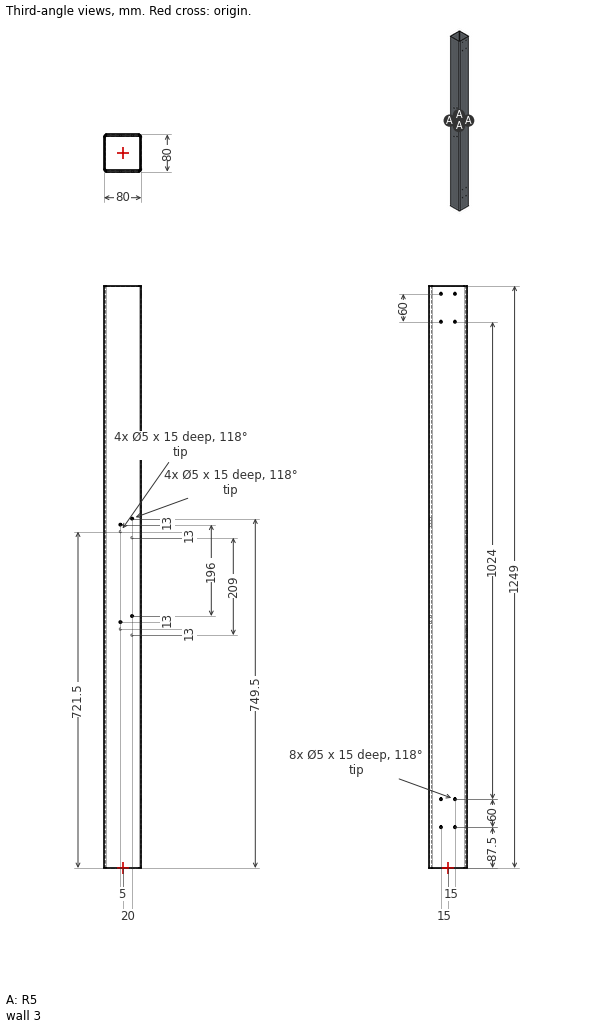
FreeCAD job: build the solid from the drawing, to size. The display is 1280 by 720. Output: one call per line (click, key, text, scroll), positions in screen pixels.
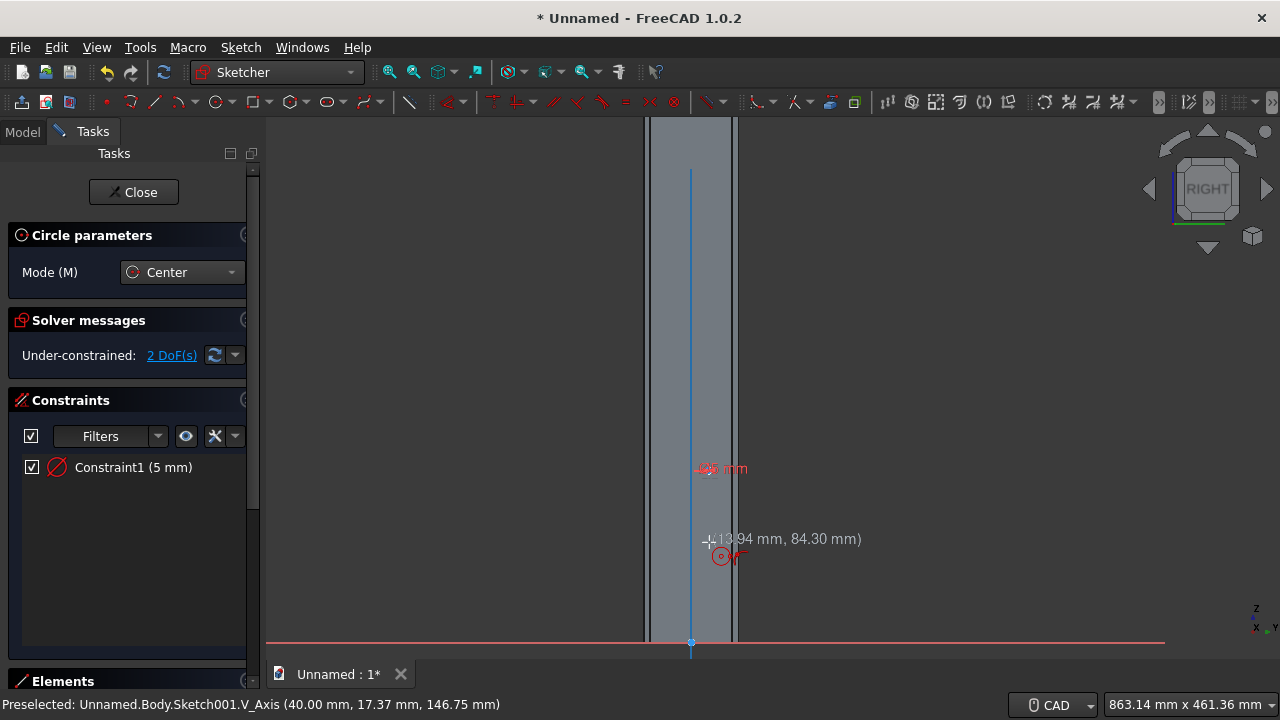
click(709, 540)
move(711, 538)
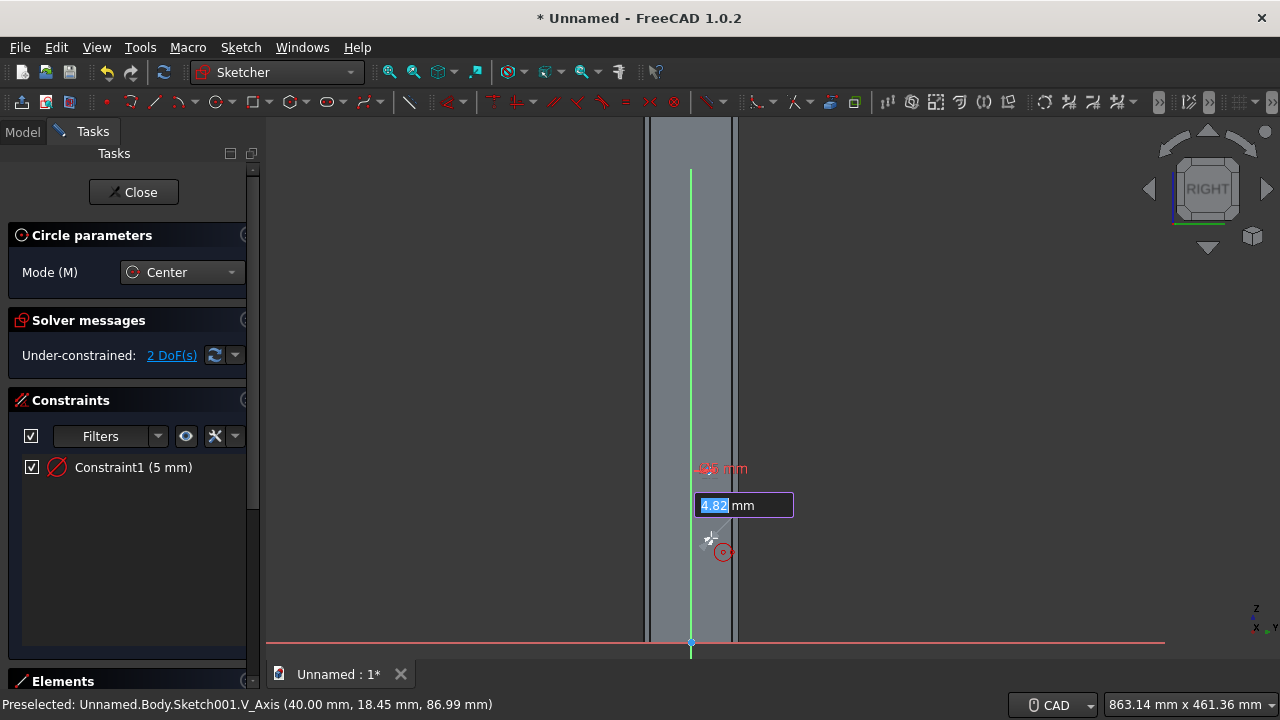
text(5)
key(Return)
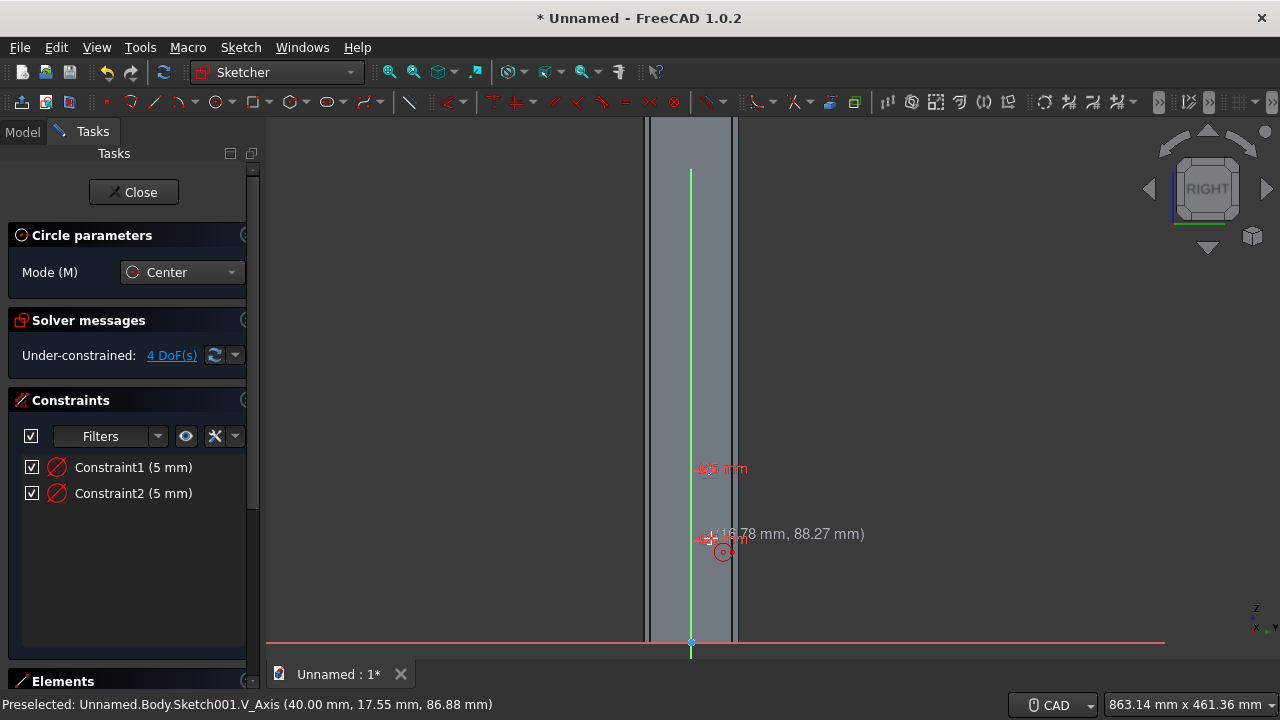
scroll(674, 540, up, 11)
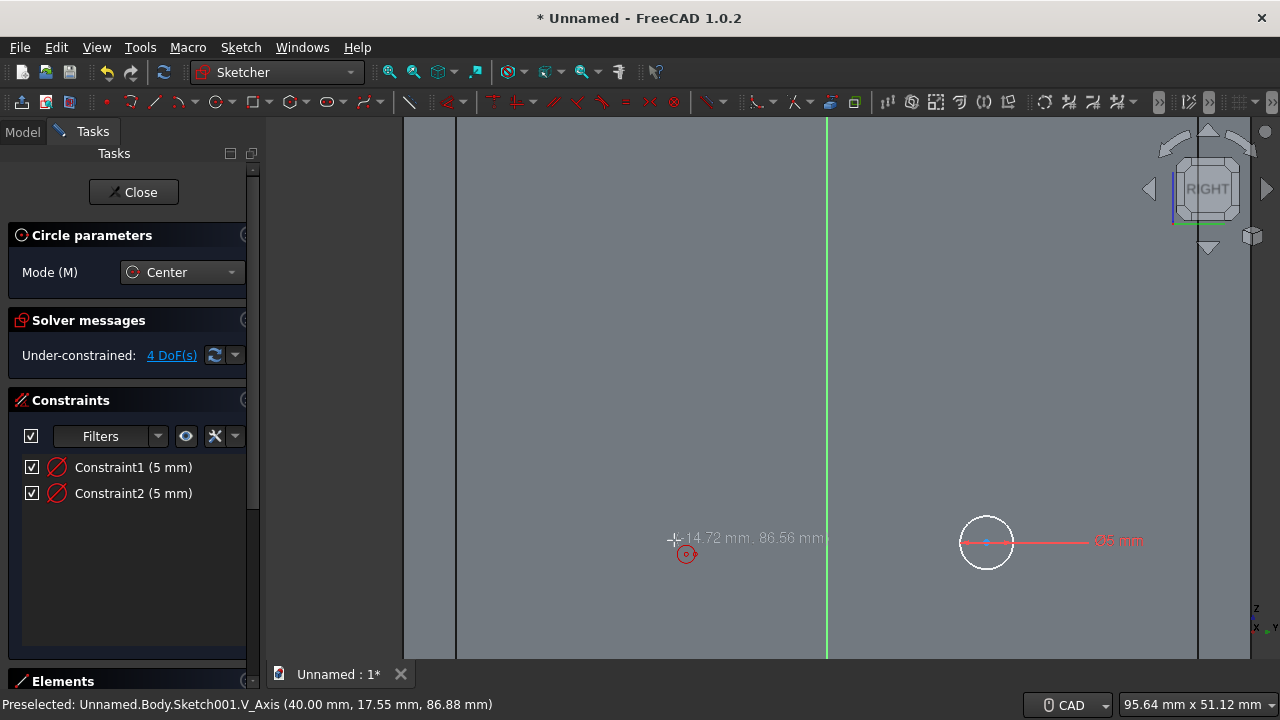
scroll(701, 542, down, 18)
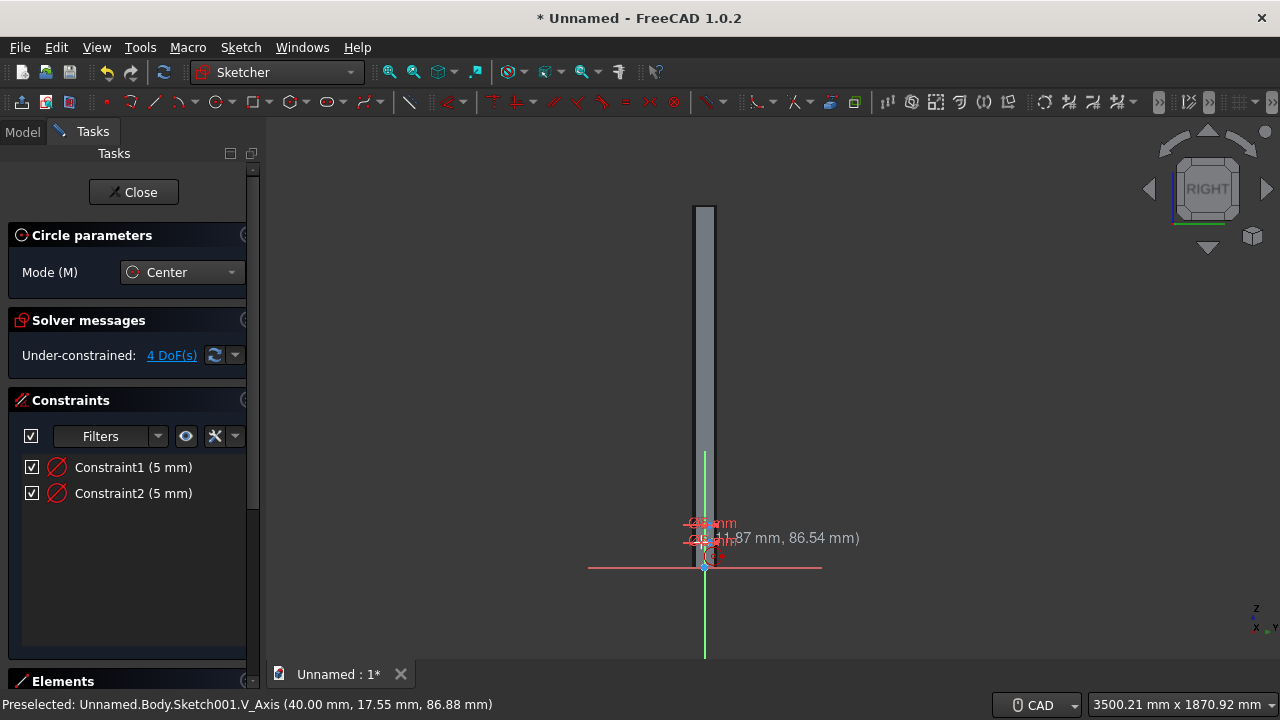
scroll(701, 543, up, 7)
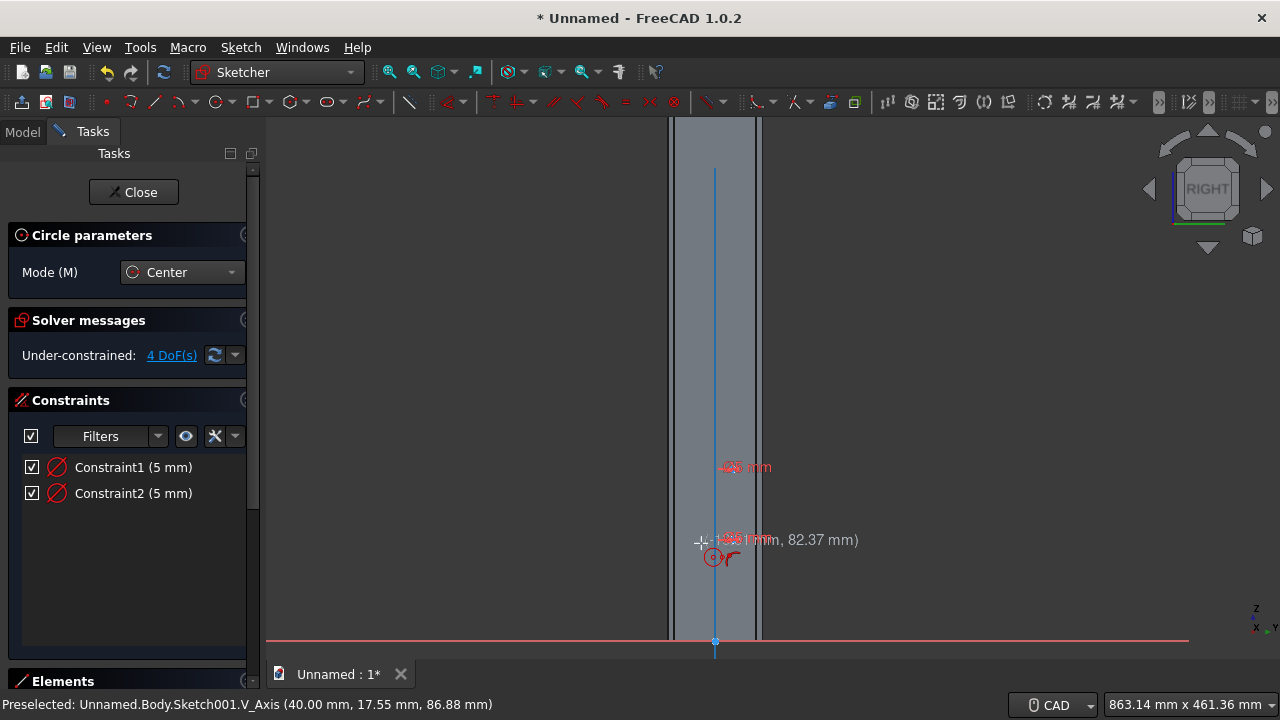
click(698, 539)
move(700, 537)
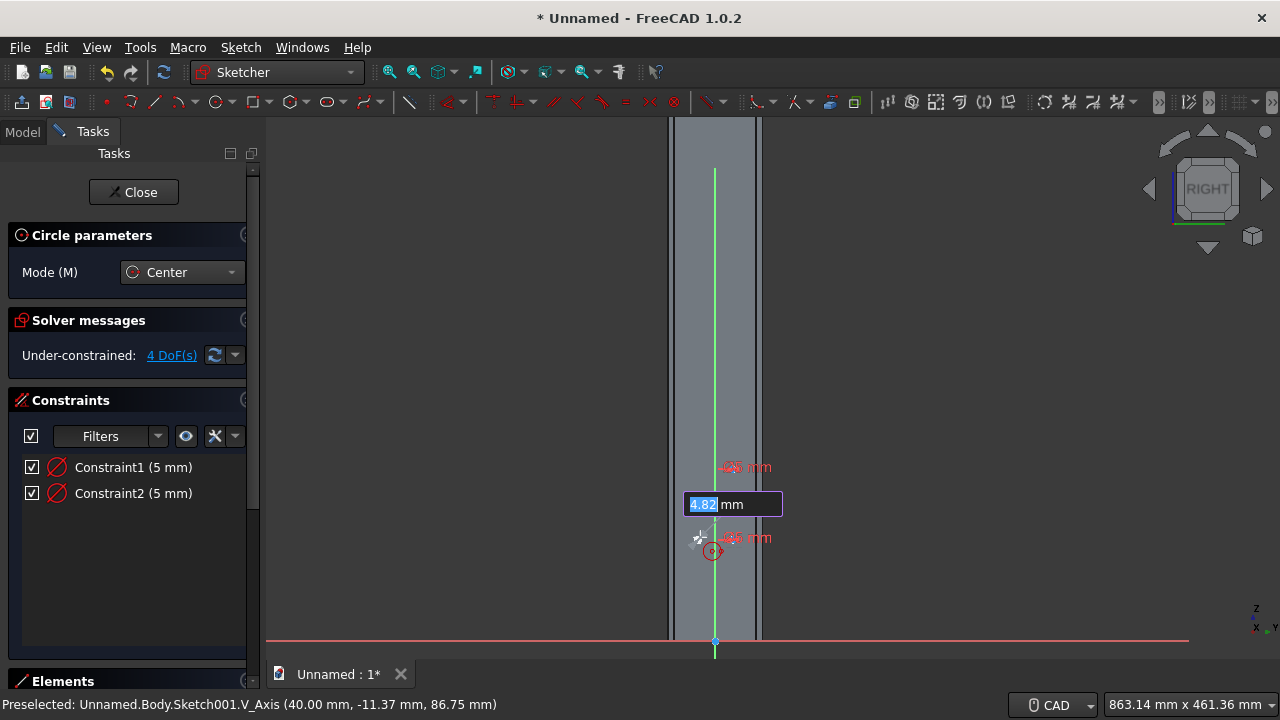
text(5)
key(Return)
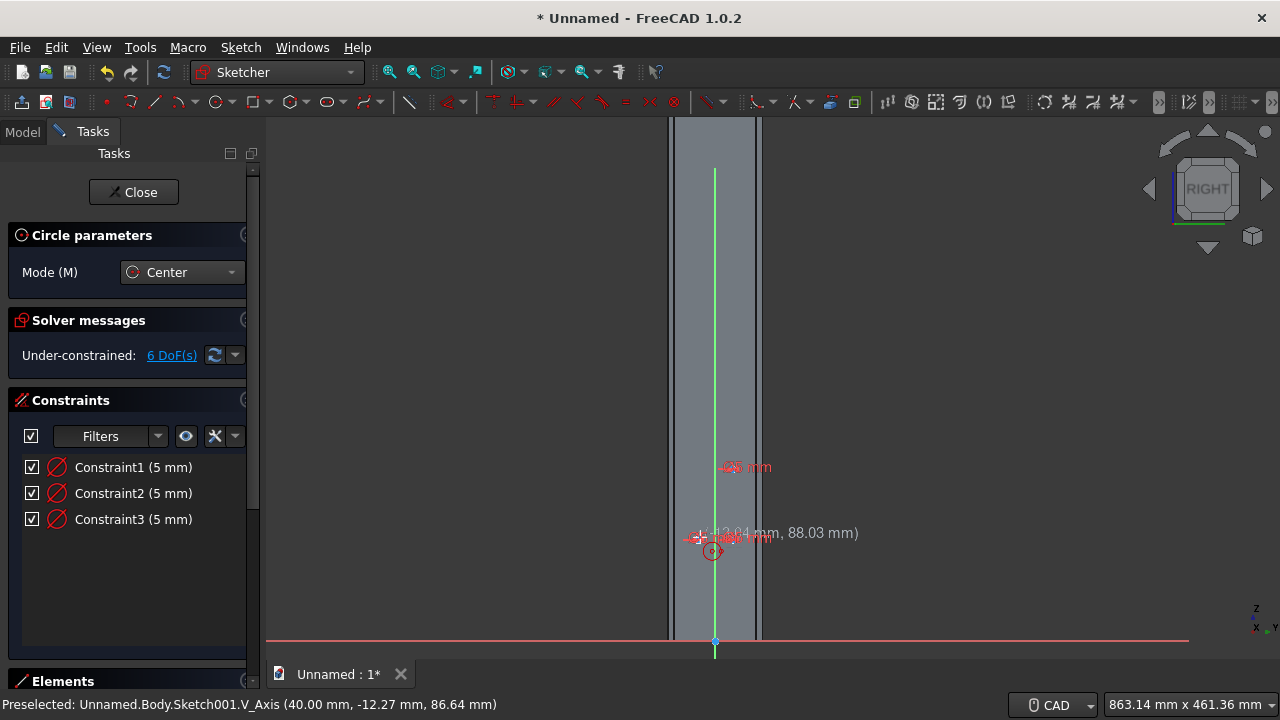
scroll(698, 468, up, 11)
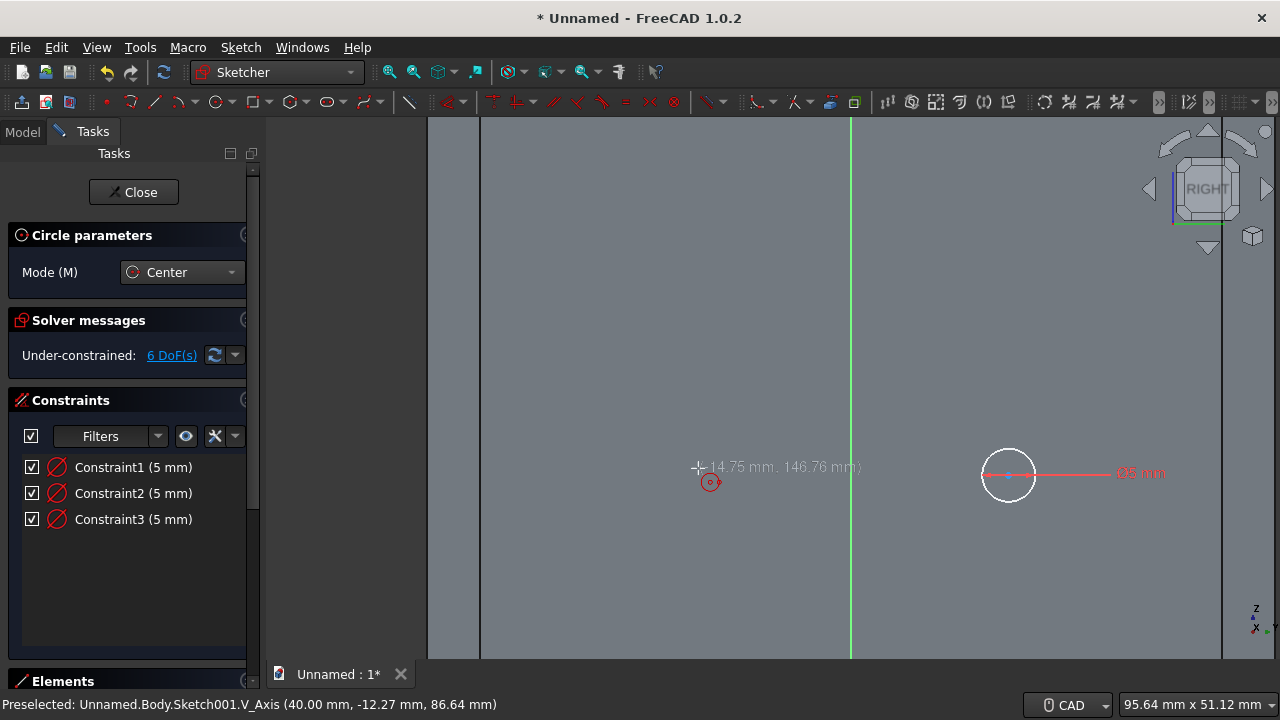
scroll(700, 526, down, 18)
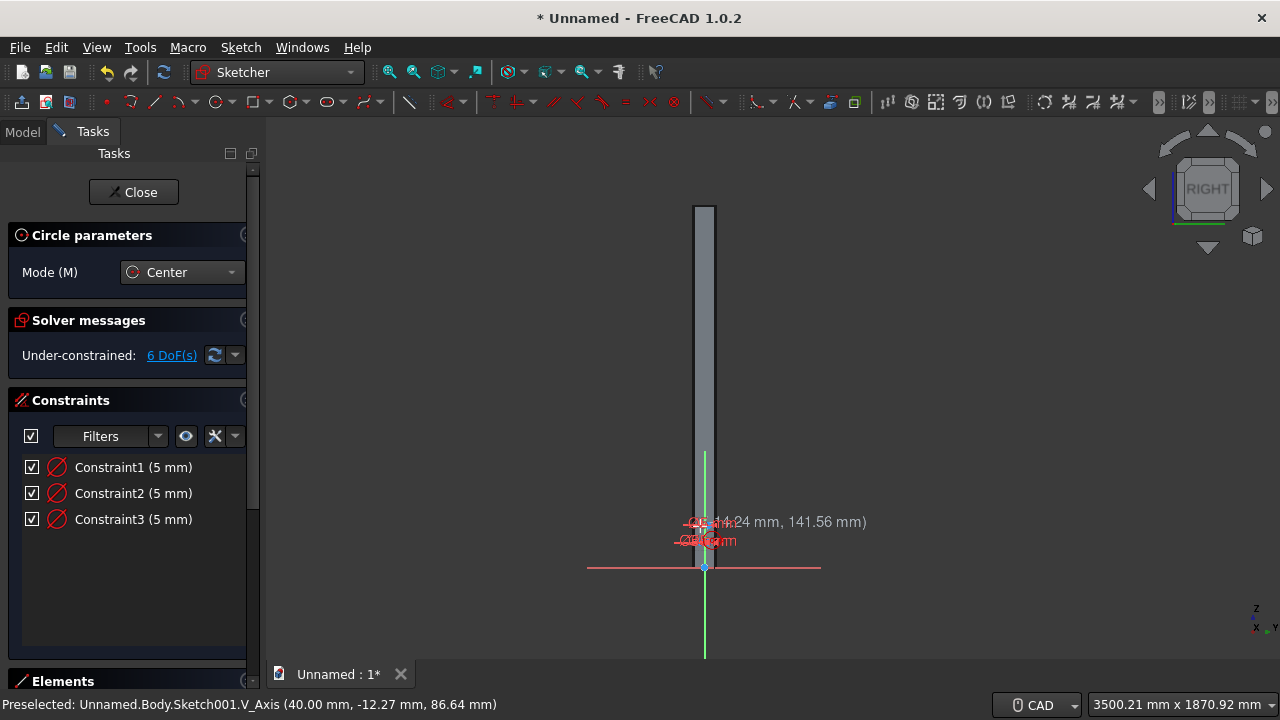
scroll(700, 525, up, 7)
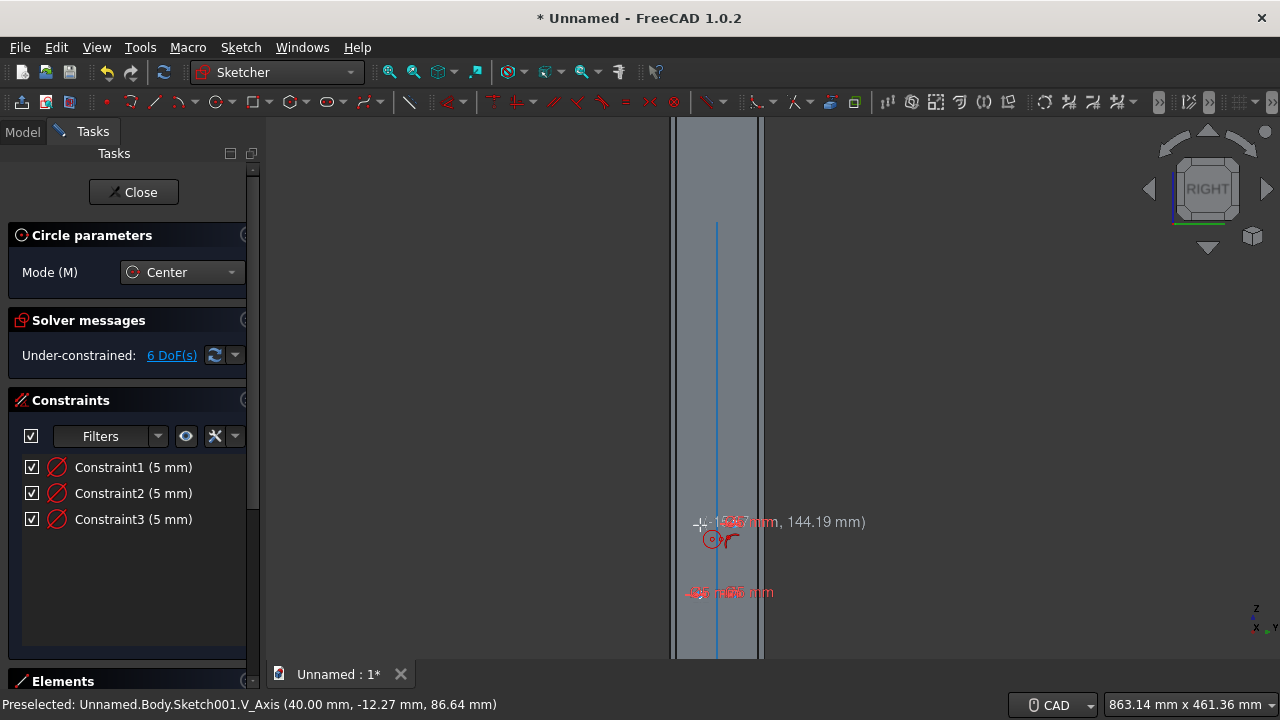
click(699, 523)
move(702, 521)